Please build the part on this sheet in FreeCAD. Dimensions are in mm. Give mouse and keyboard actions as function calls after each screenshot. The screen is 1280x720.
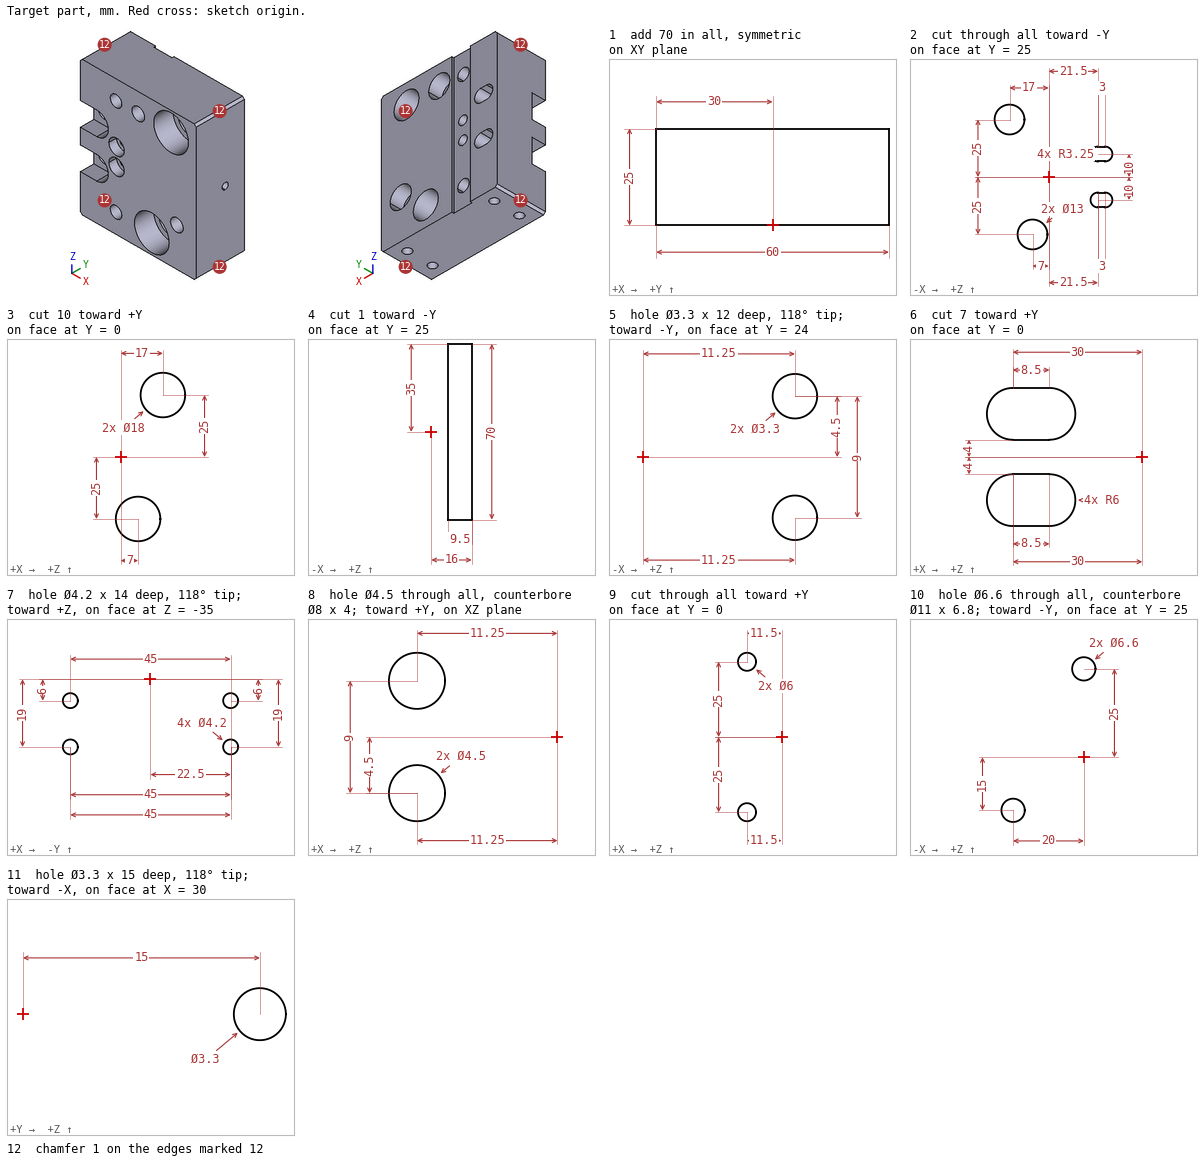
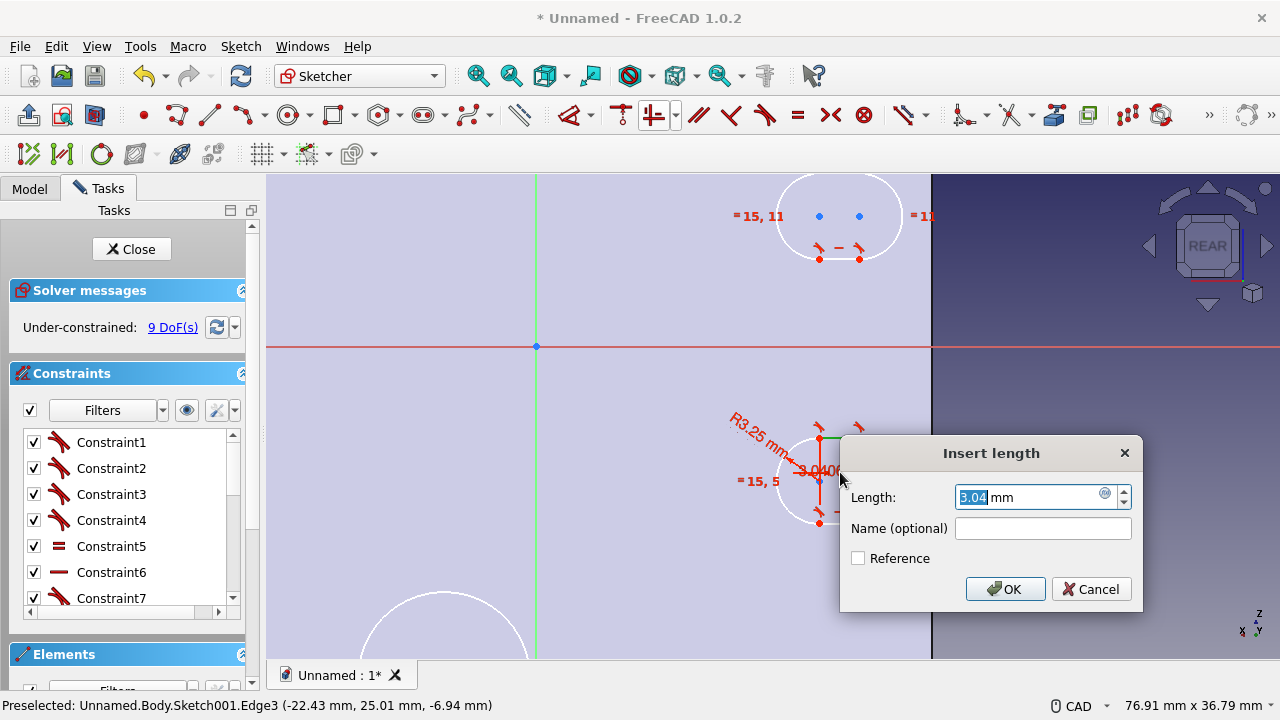
text(3)
key(Return)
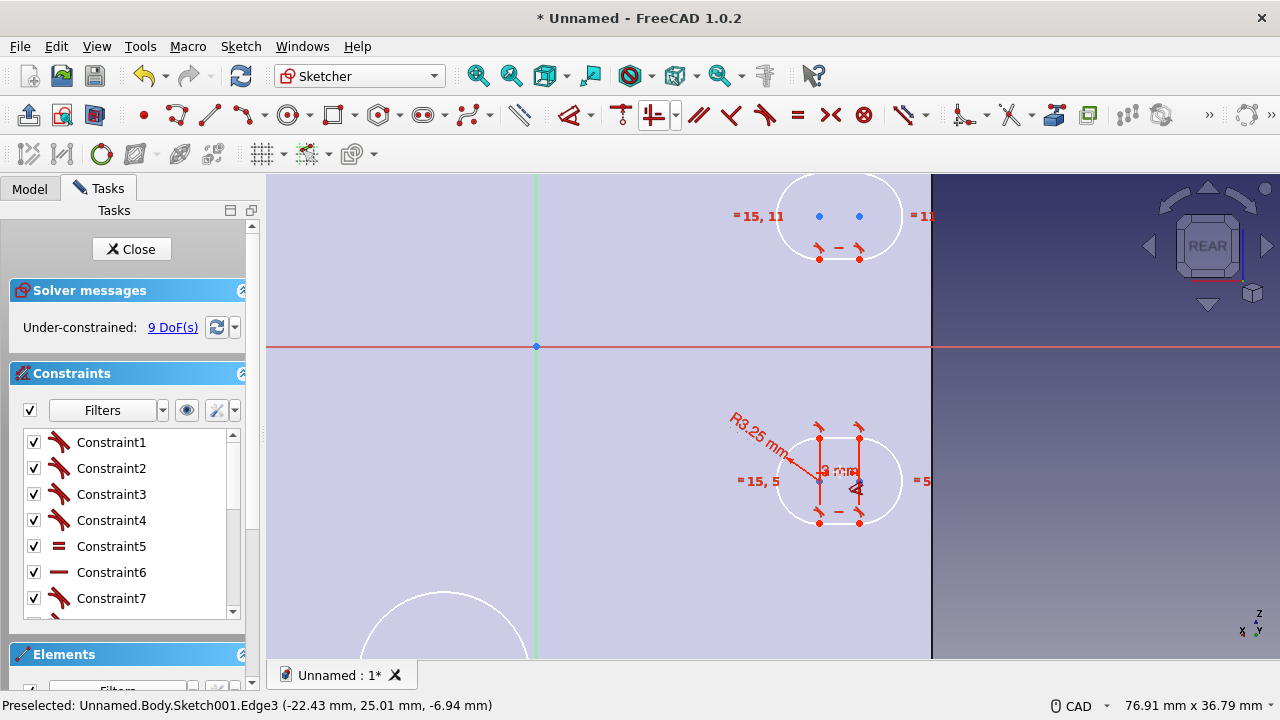
scroll(786, 457, down, 5)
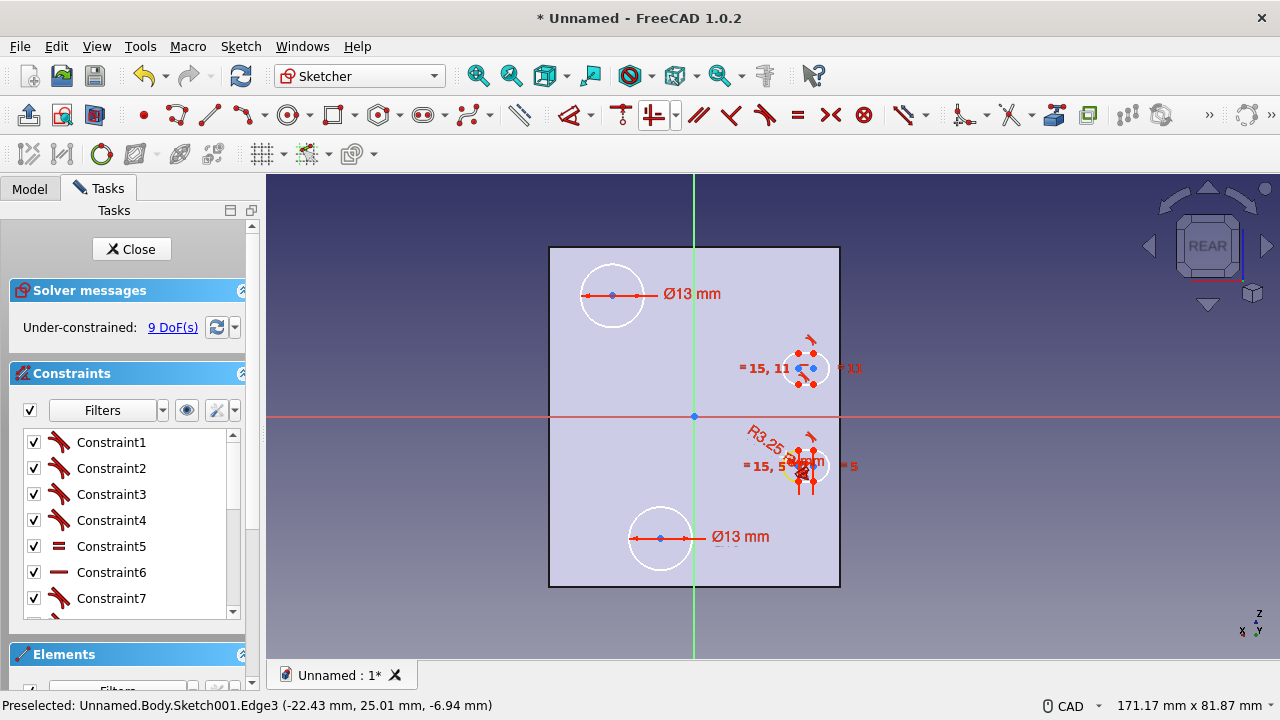
scroll(803, 353, up, 6)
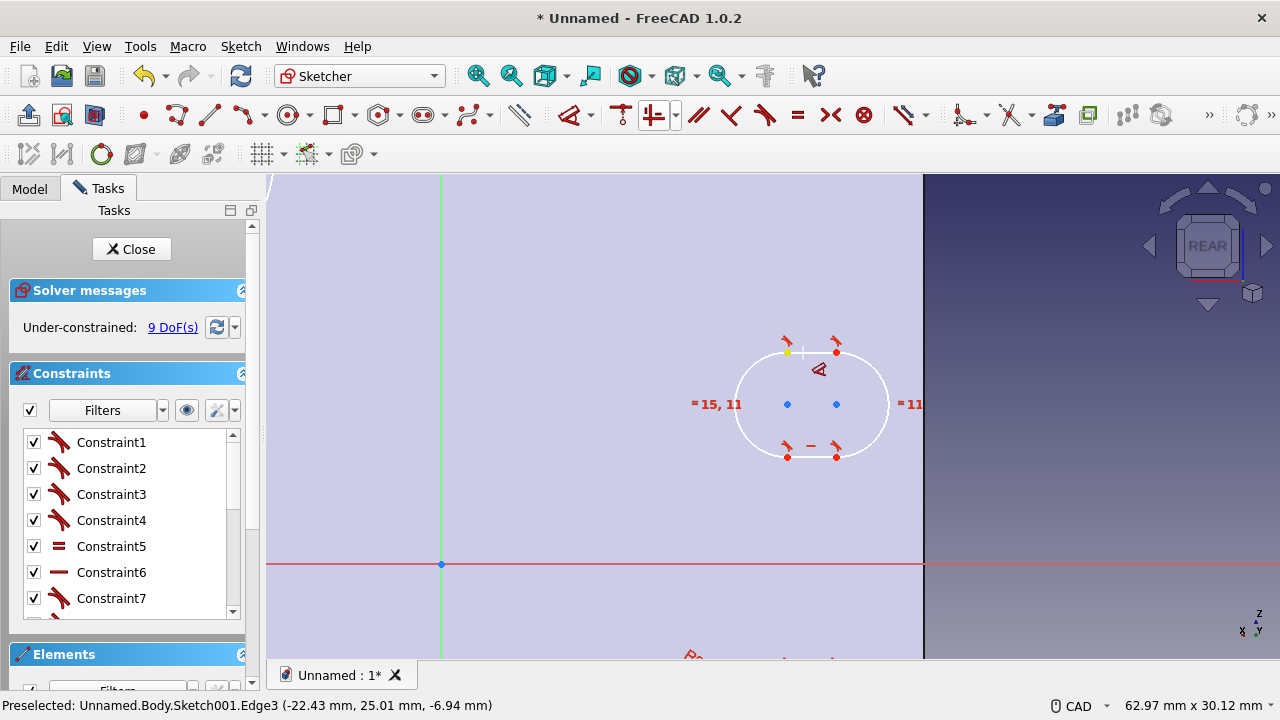
click(802, 353)
click(812, 319)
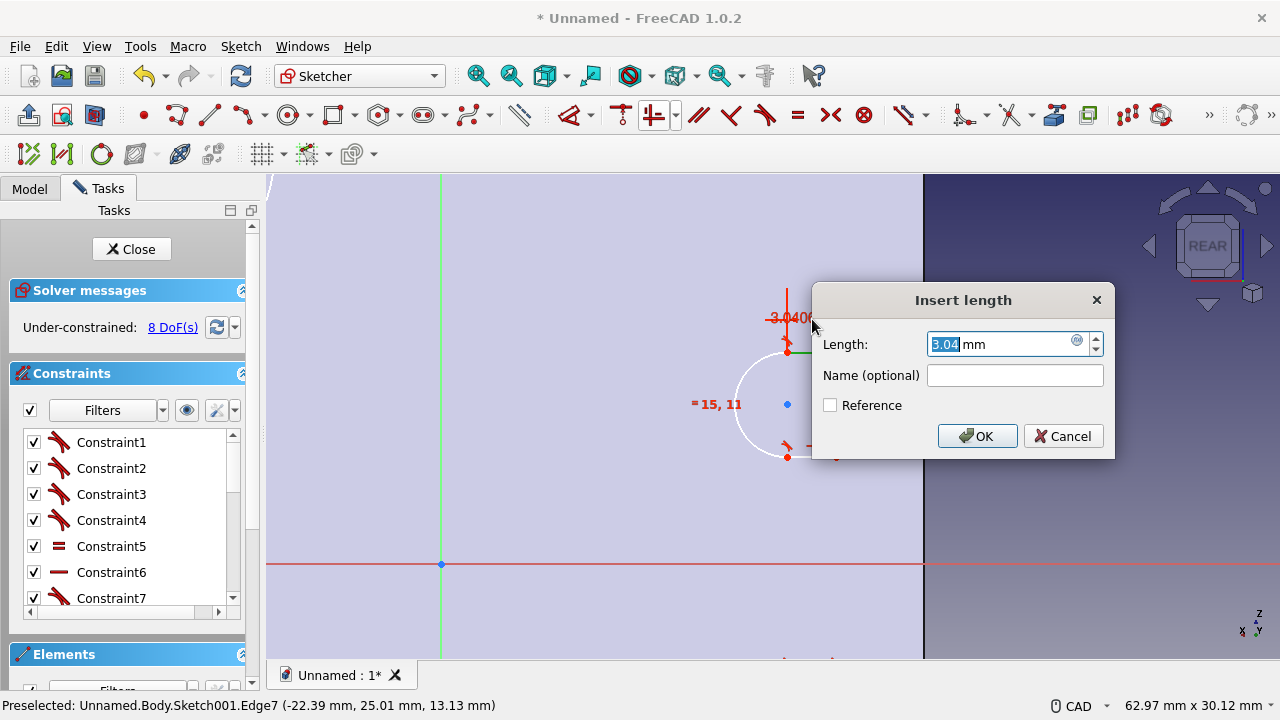
text(3)
key(Return)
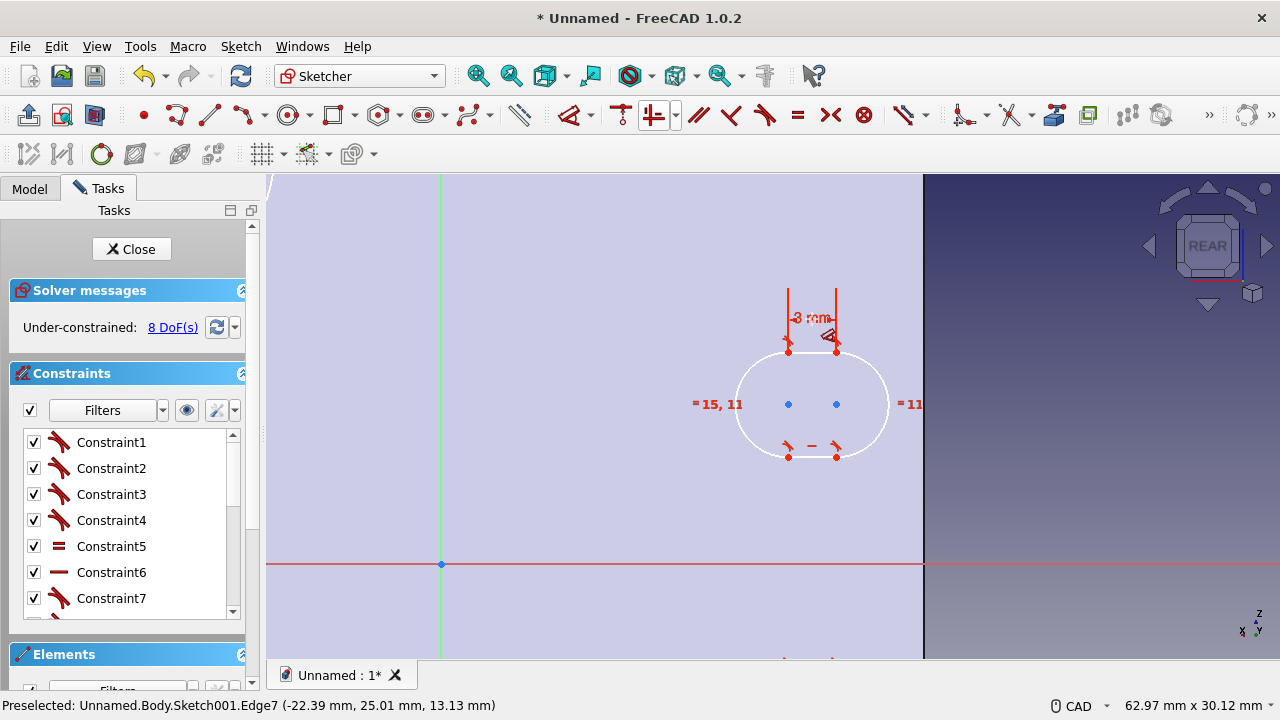
scroll(803, 353, down, 6)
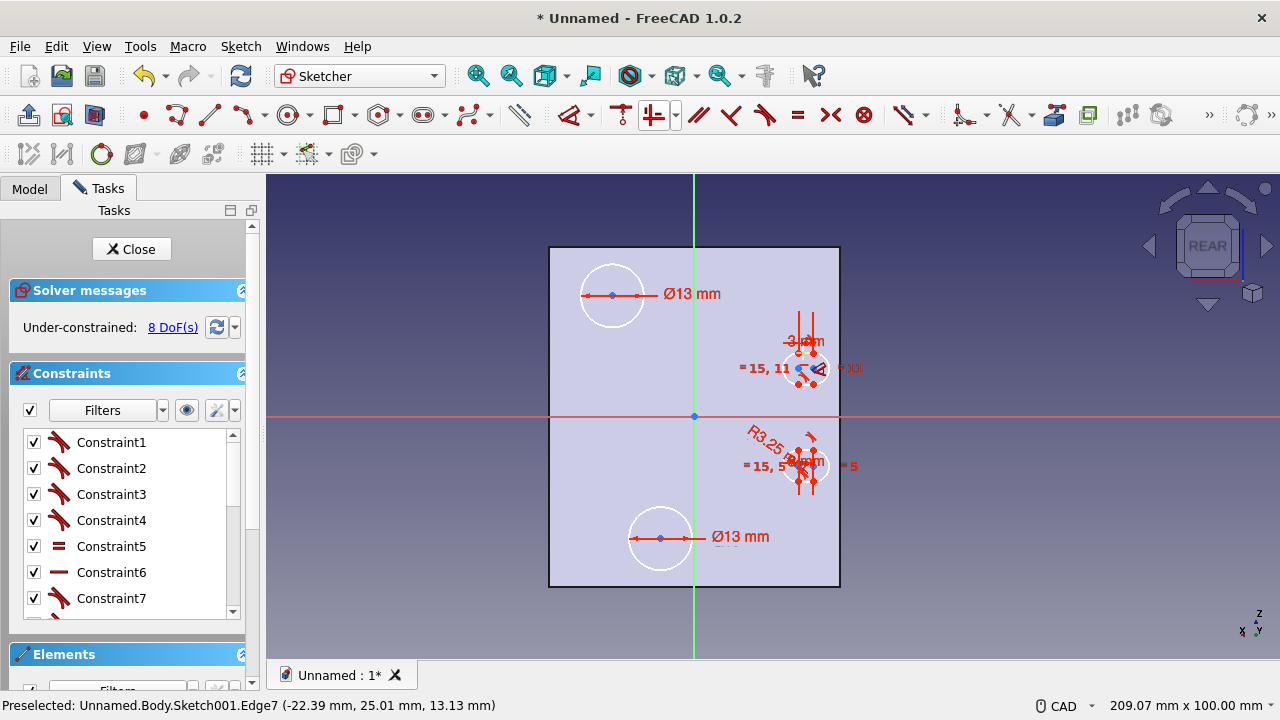
click(661, 539)
click(678, 383)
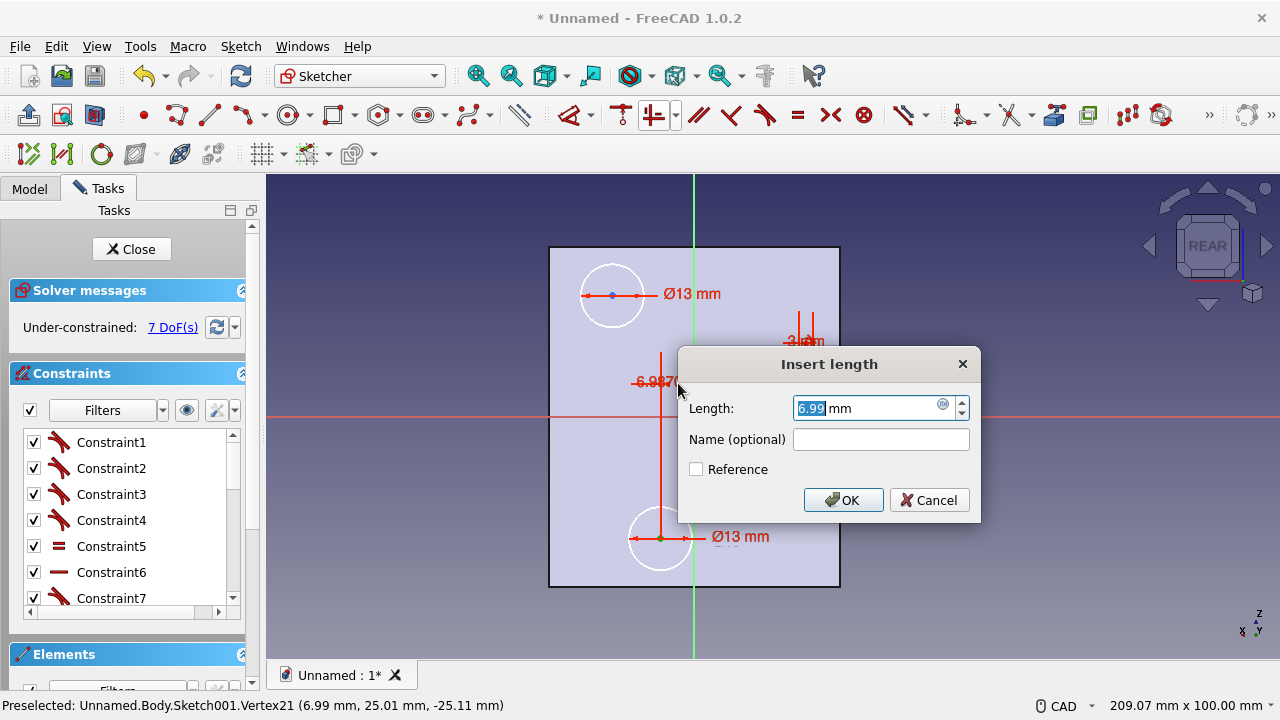
text(7)
key(Return)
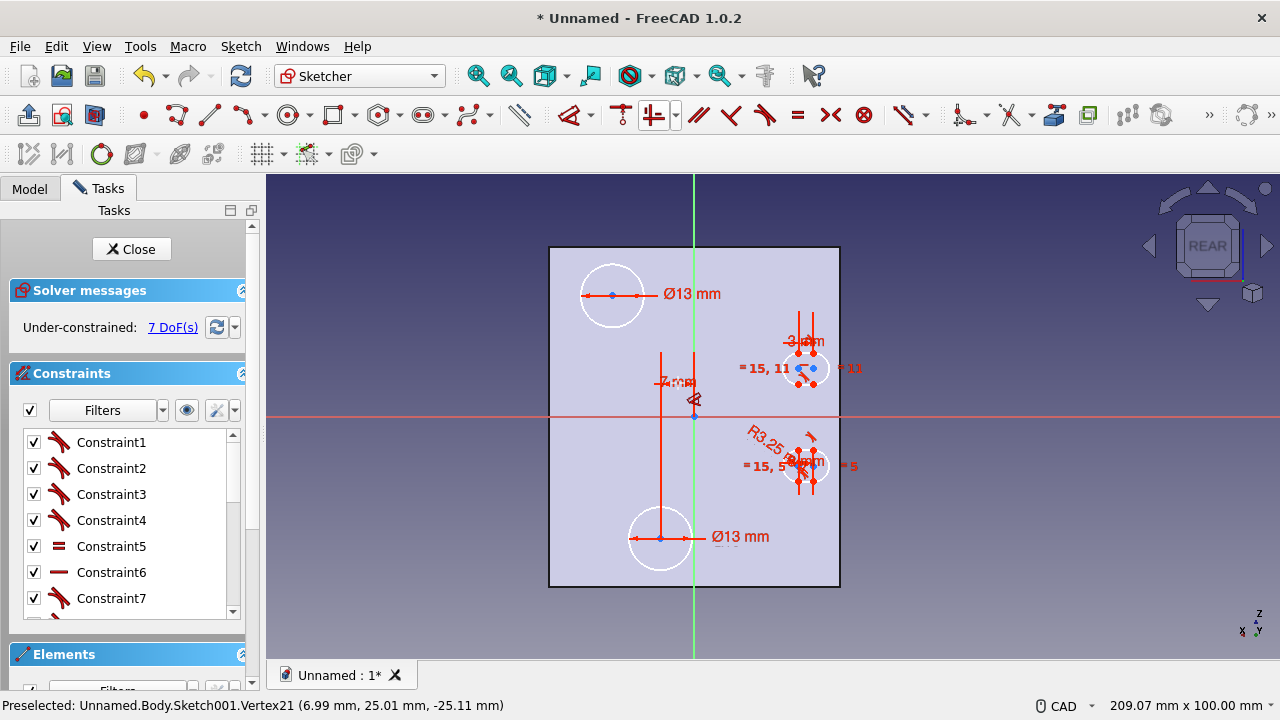
click(661, 539)
click(627, 478)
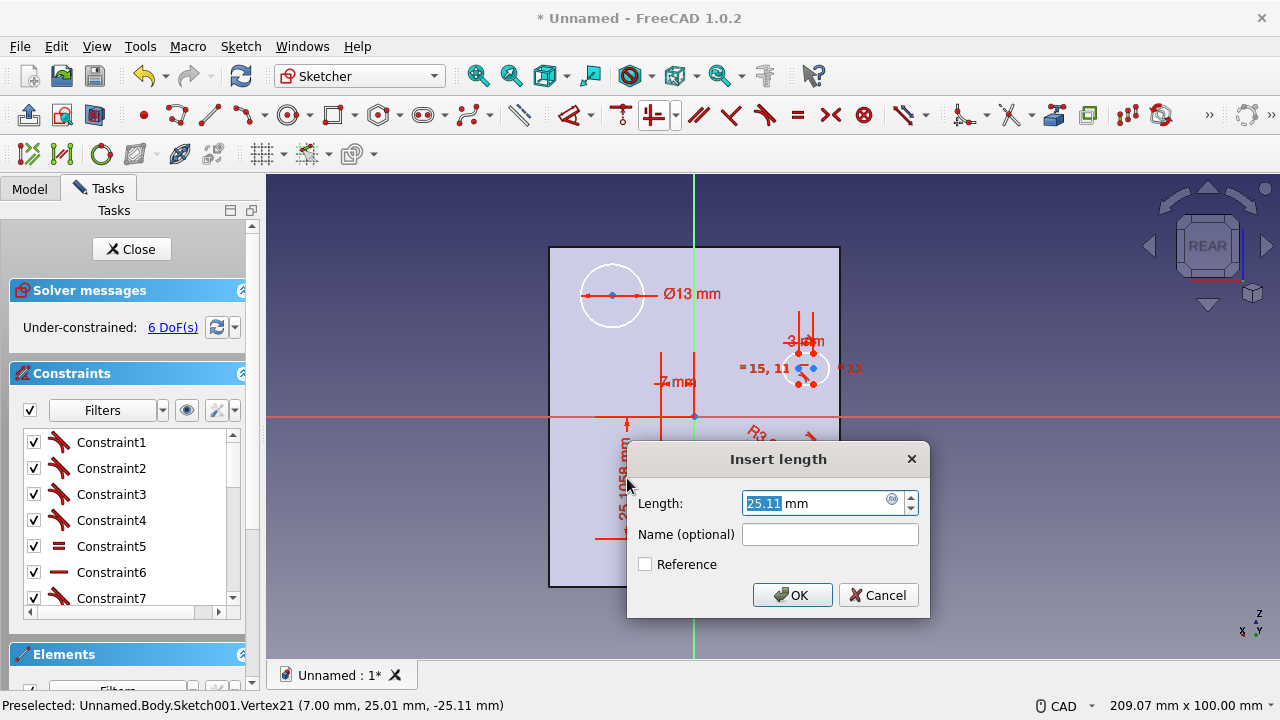
text(25)
key(Return)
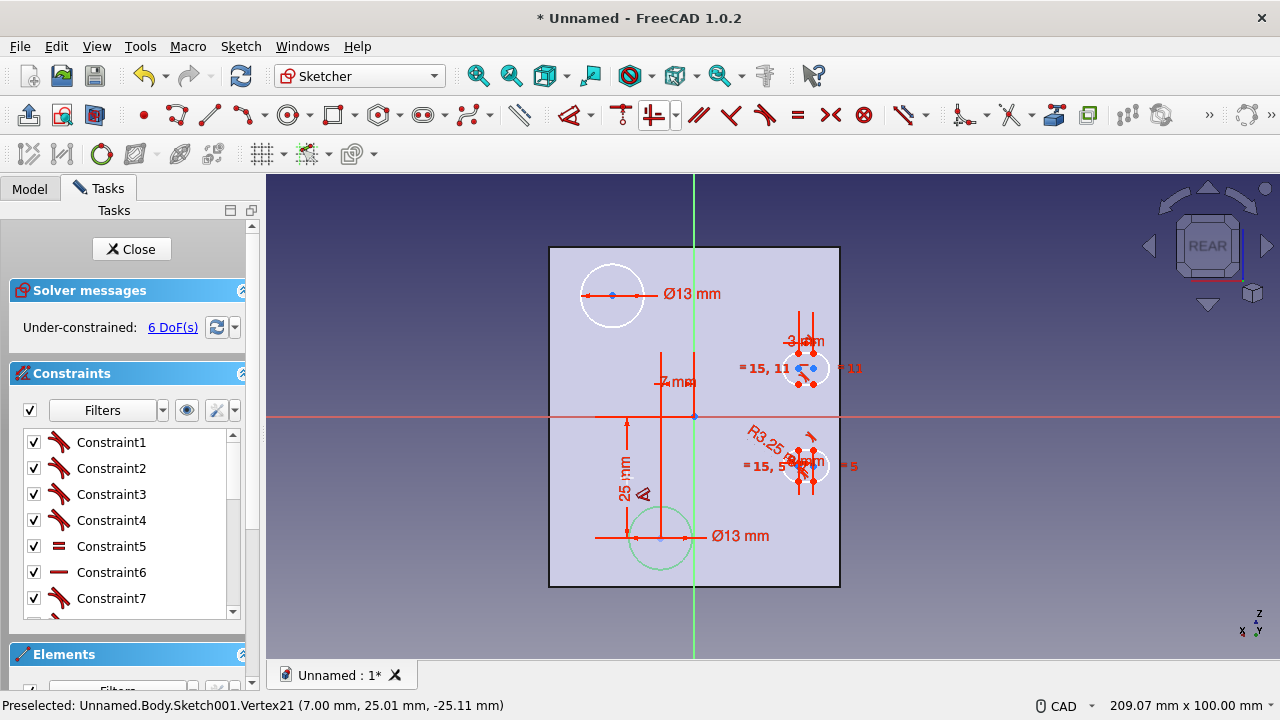
click(612, 296)
click(653, 262)